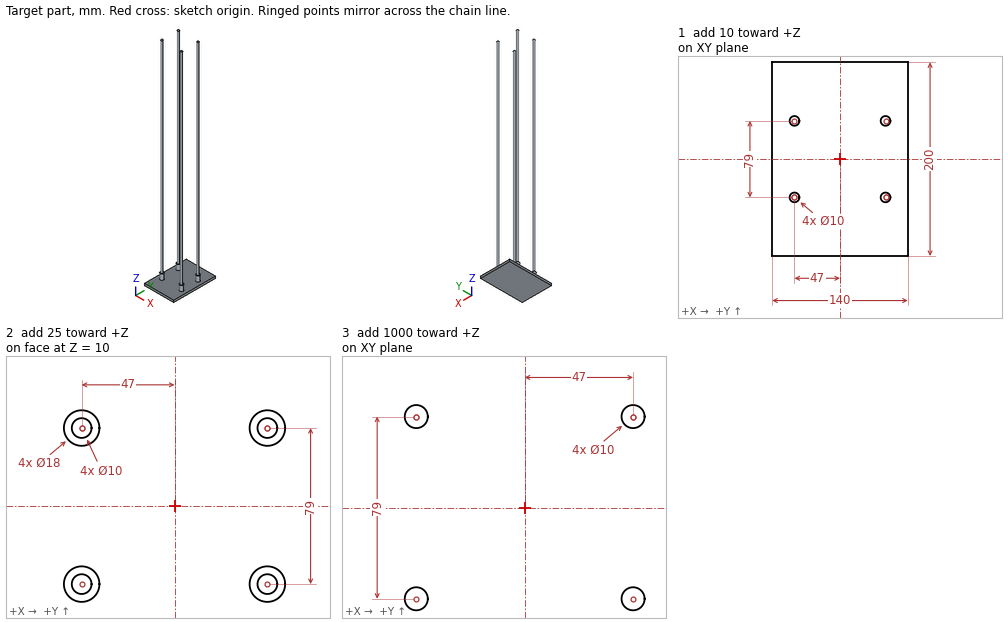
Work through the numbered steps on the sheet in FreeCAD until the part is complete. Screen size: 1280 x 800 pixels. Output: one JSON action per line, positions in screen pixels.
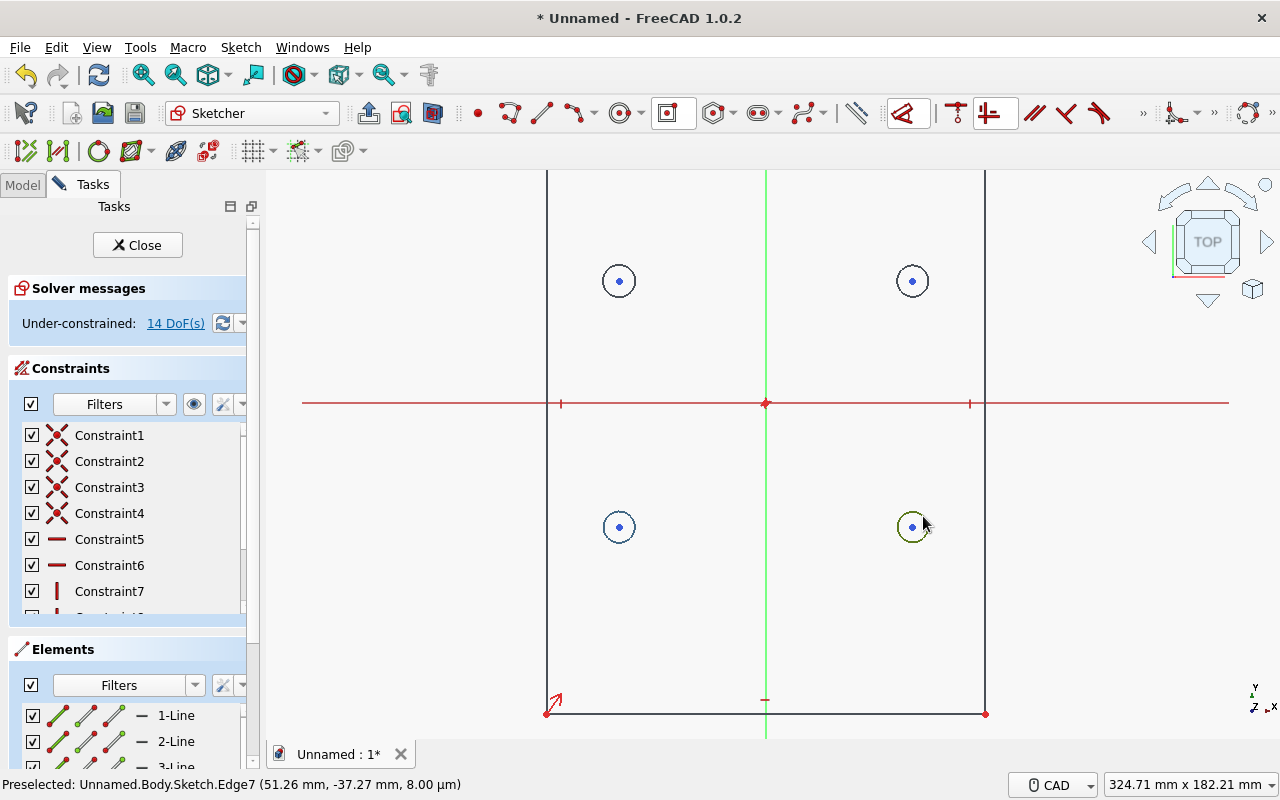
{"action": "left_click", "coordinate": [631, 270]}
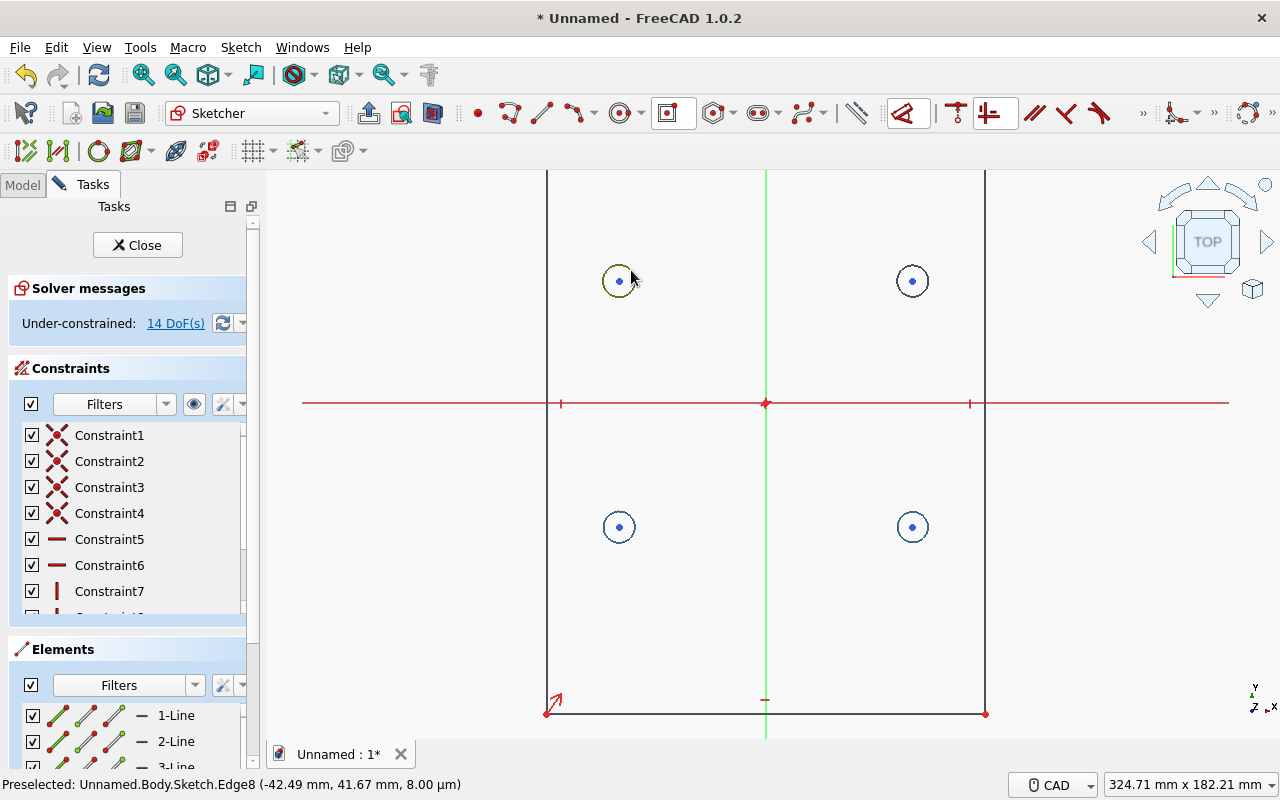
{"action": "left_click", "coordinate": [924, 270]}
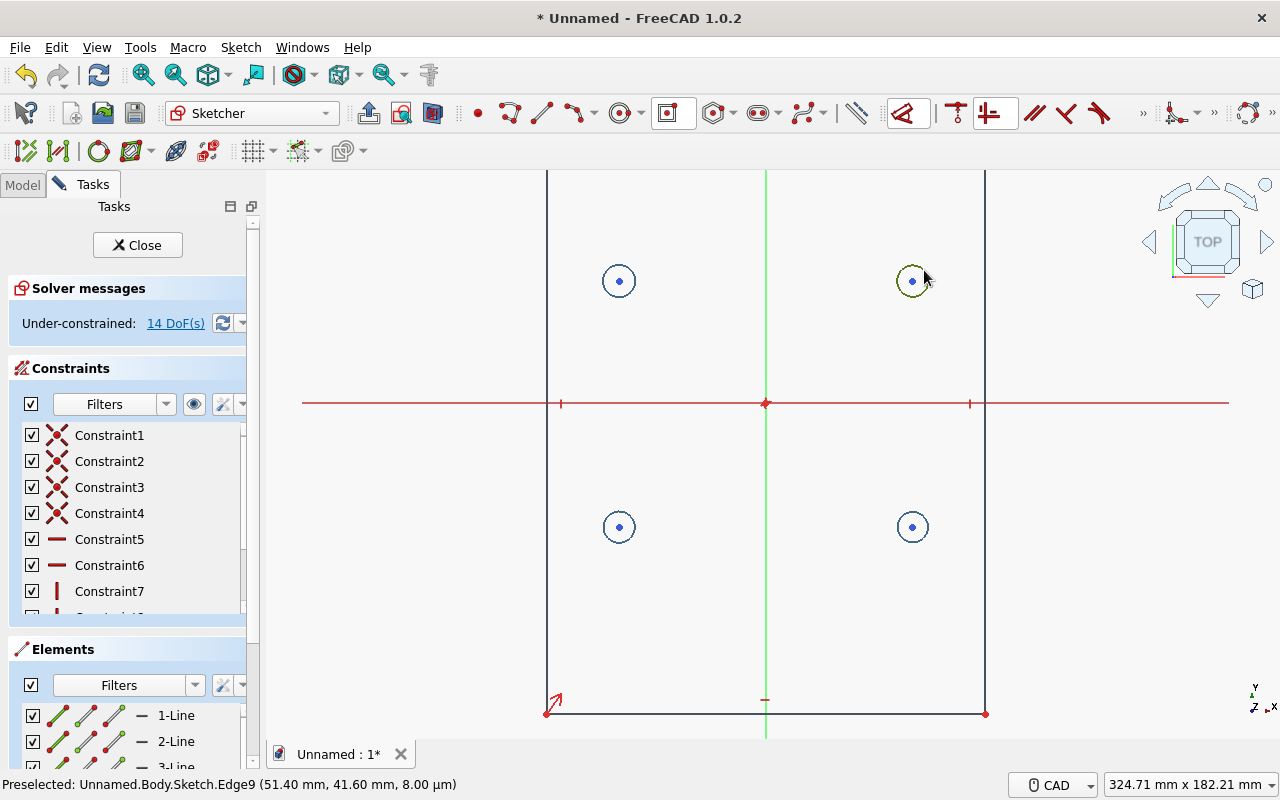
{"action": "key", "text": "e"}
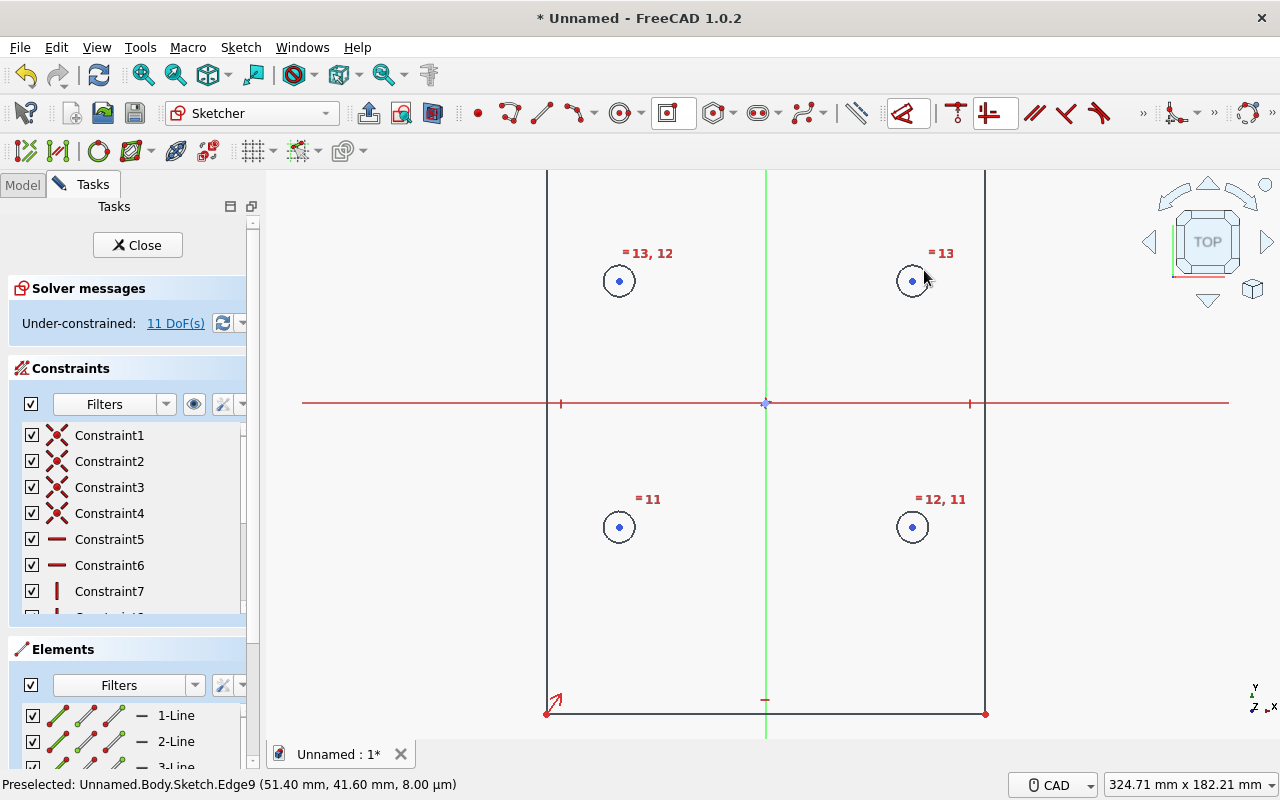
{"action": "left_click", "coordinate": [619, 527]}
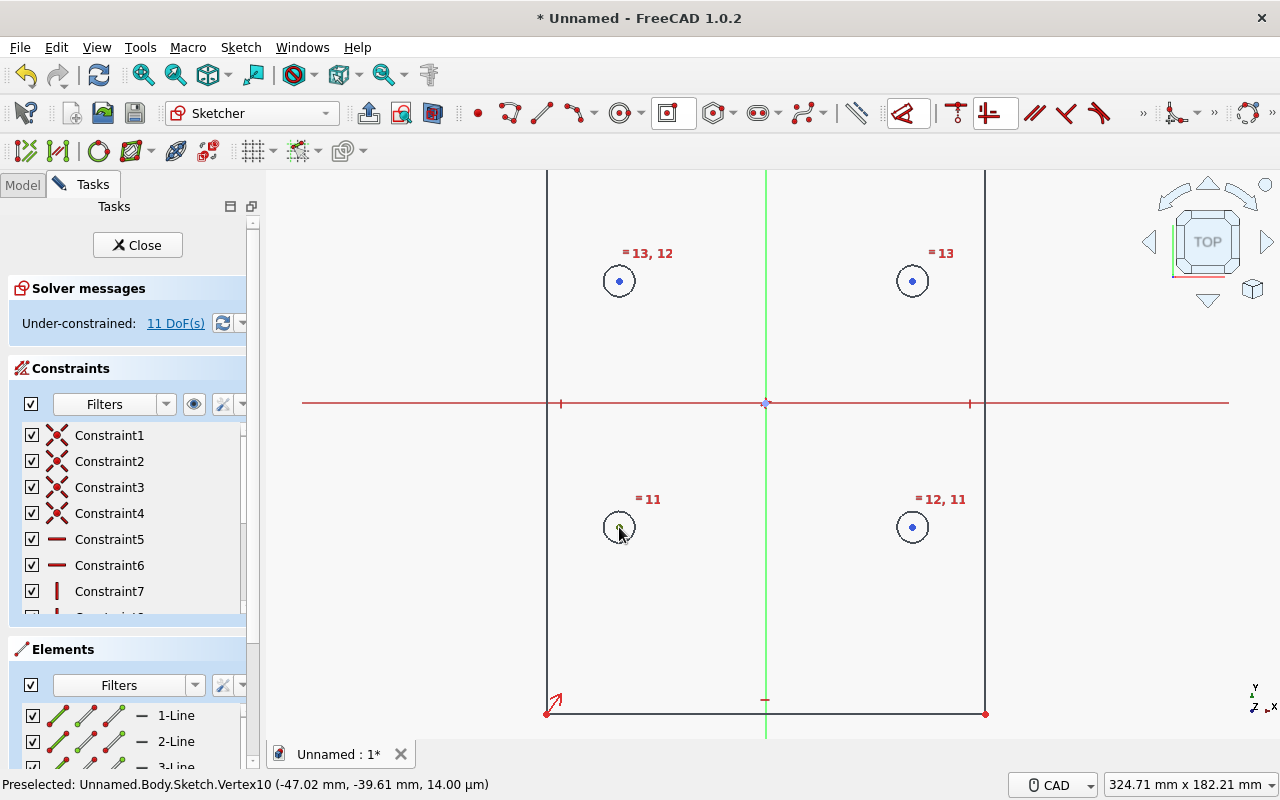
{"action": "left_click", "coordinate": [913, 527]}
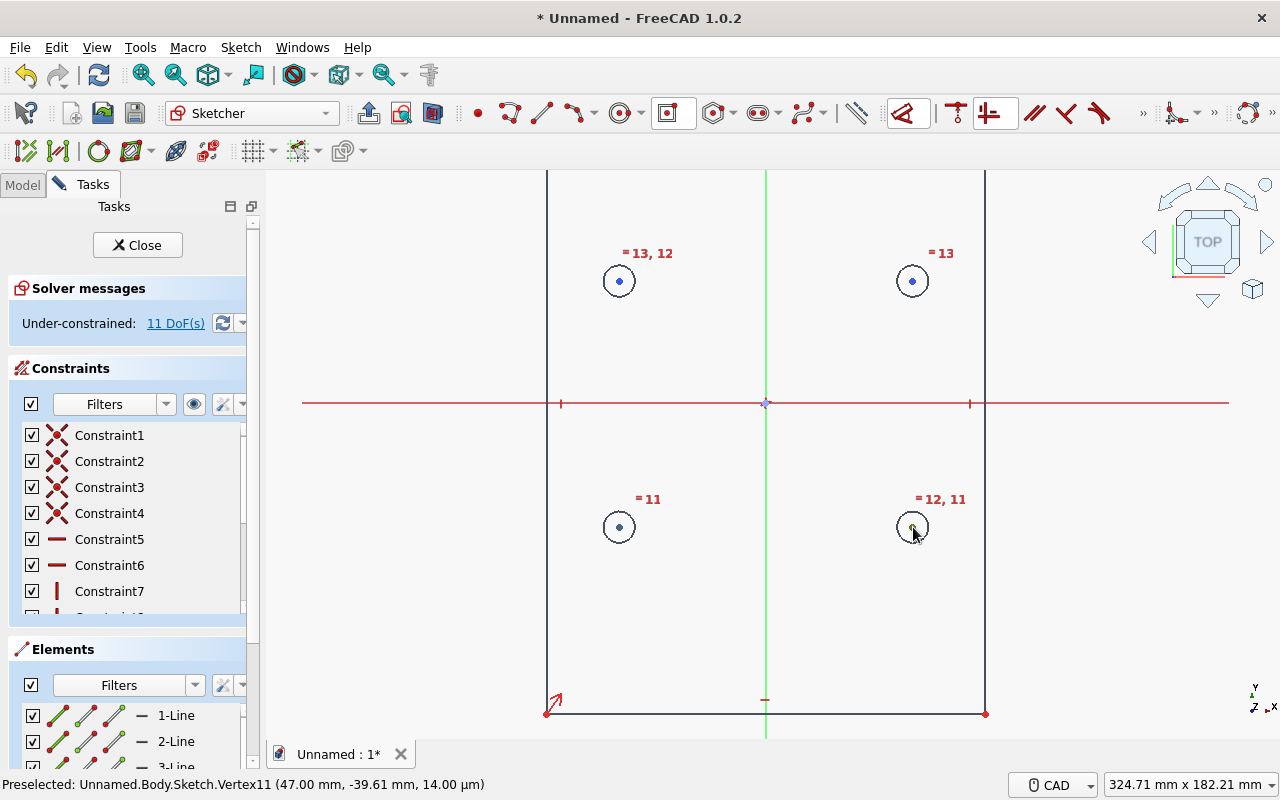
{"action": "left_click", "coordinate": [766, 674]}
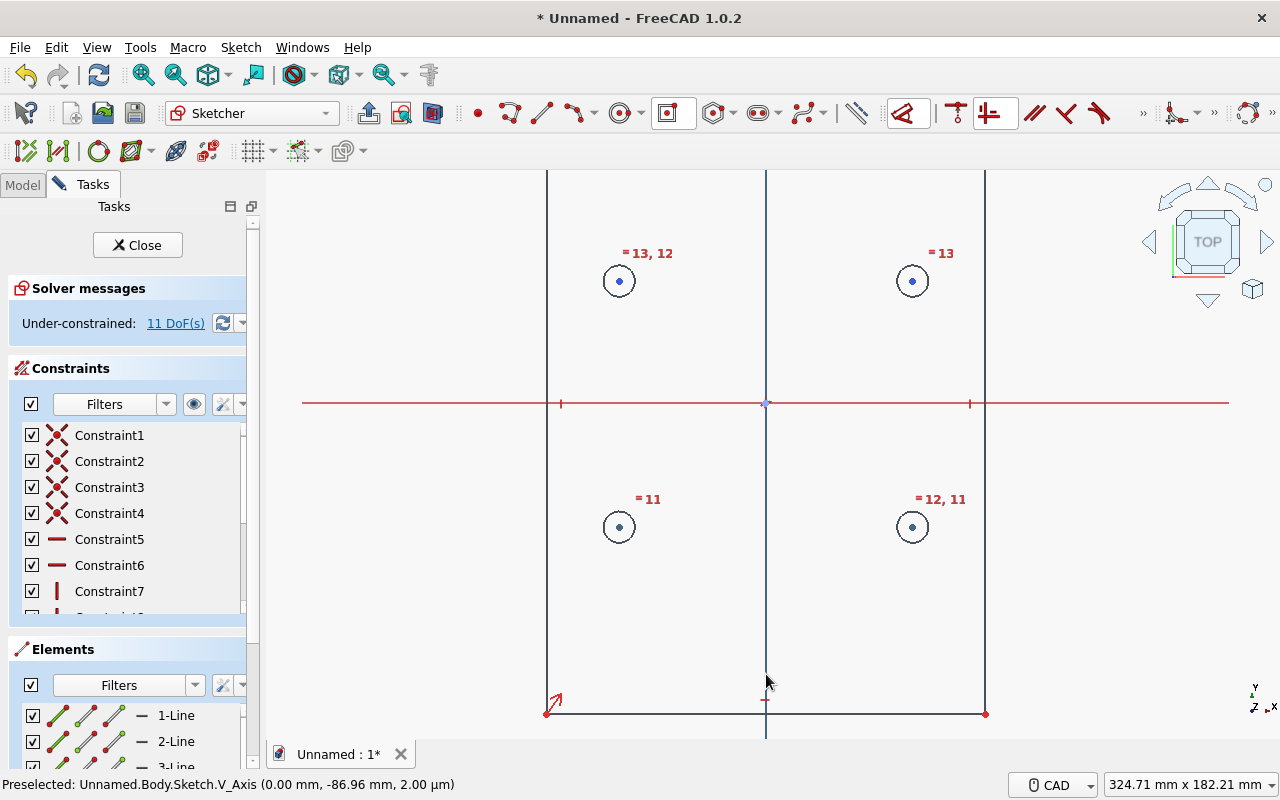
{"action": "key", "text": "s"}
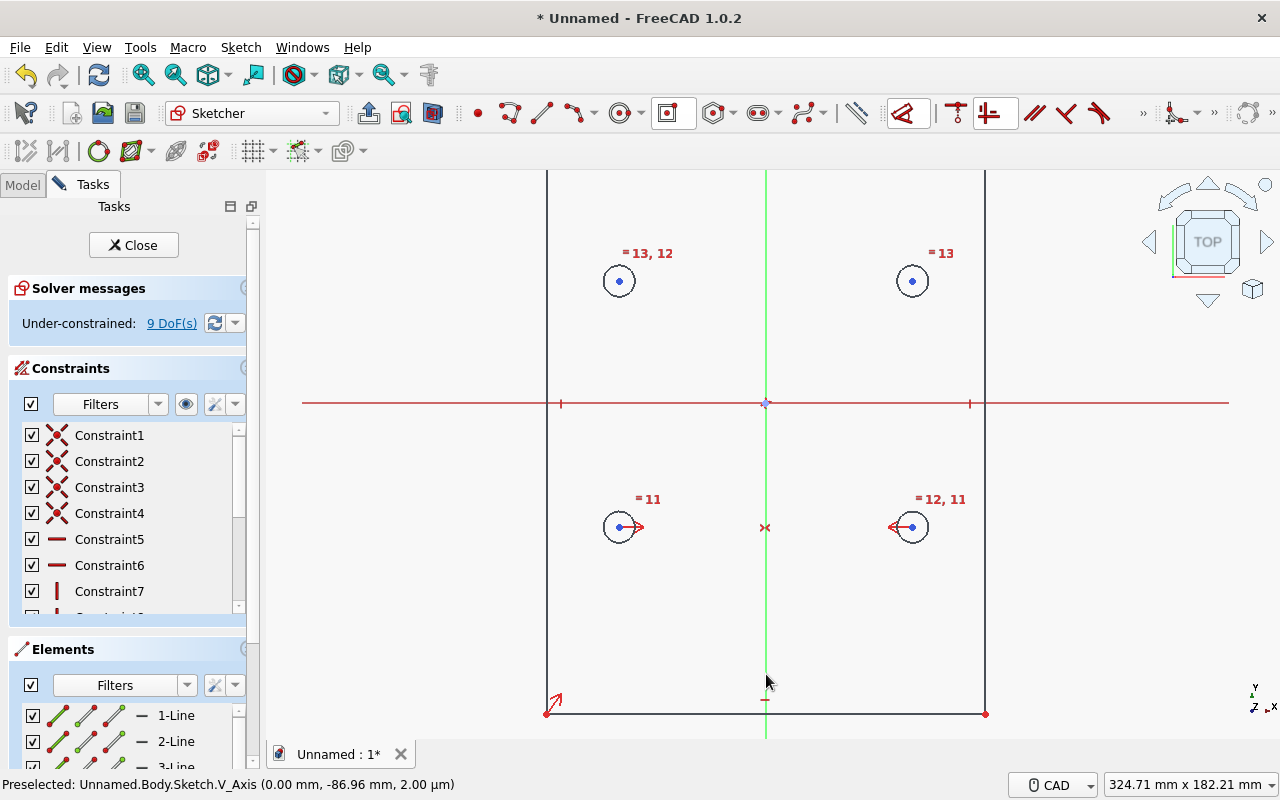
{"action": "left_click", "coordinate": [619, 527]}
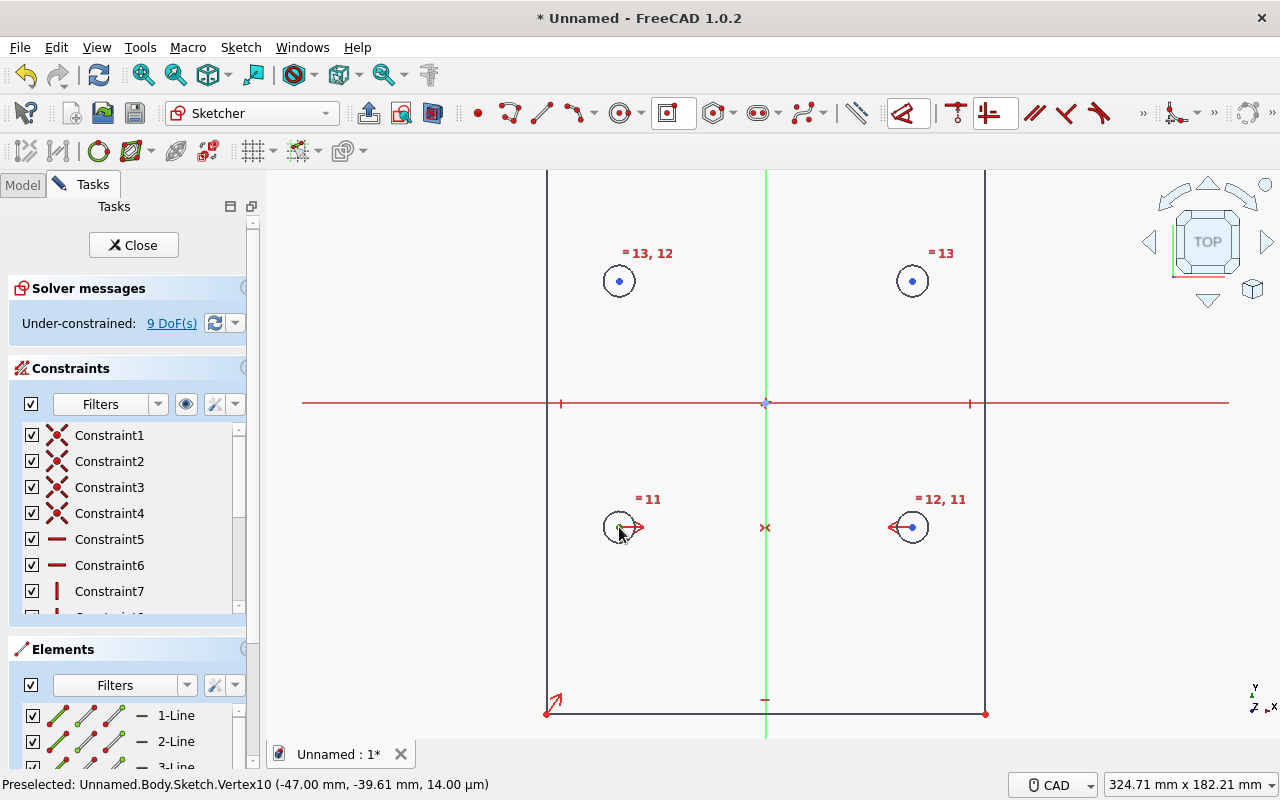
{"action": "left_click", "coordinate": [619, 281]}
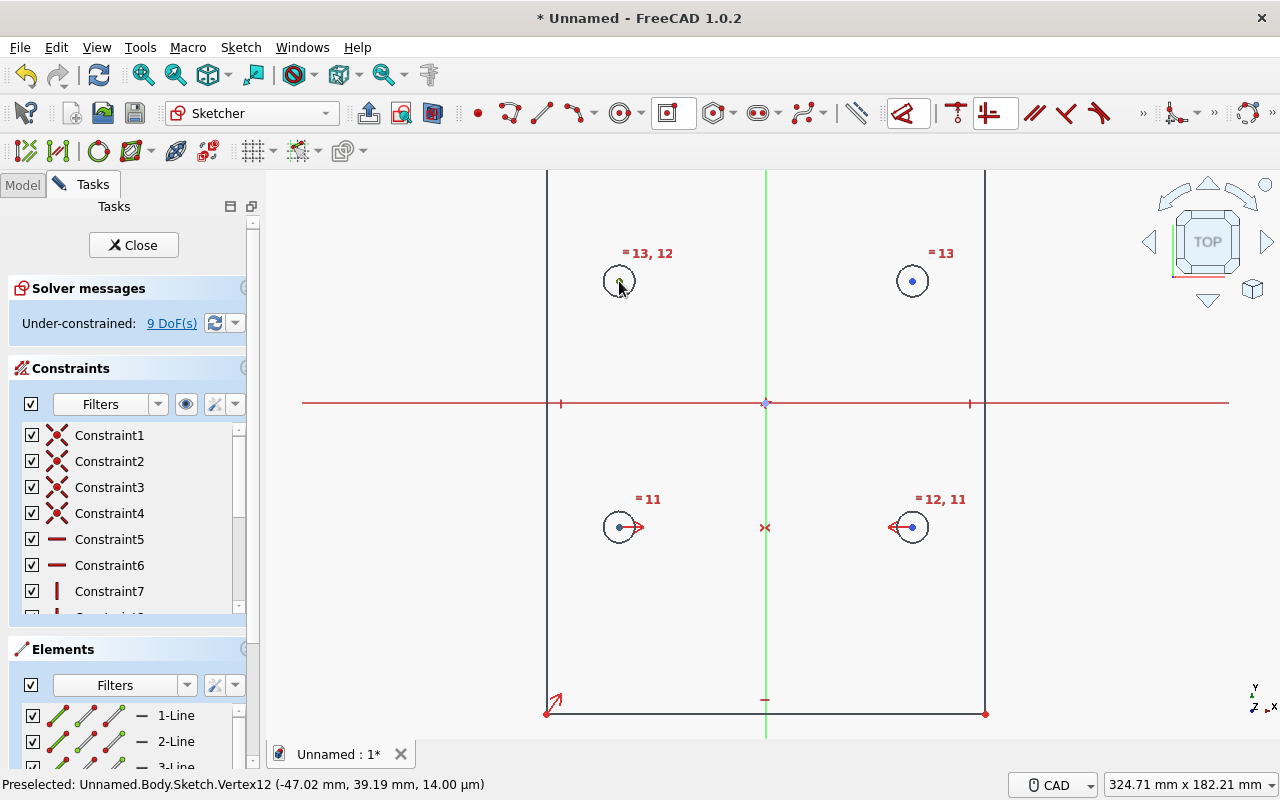
{"action": "left_click", "coordinate": [353, 403]}